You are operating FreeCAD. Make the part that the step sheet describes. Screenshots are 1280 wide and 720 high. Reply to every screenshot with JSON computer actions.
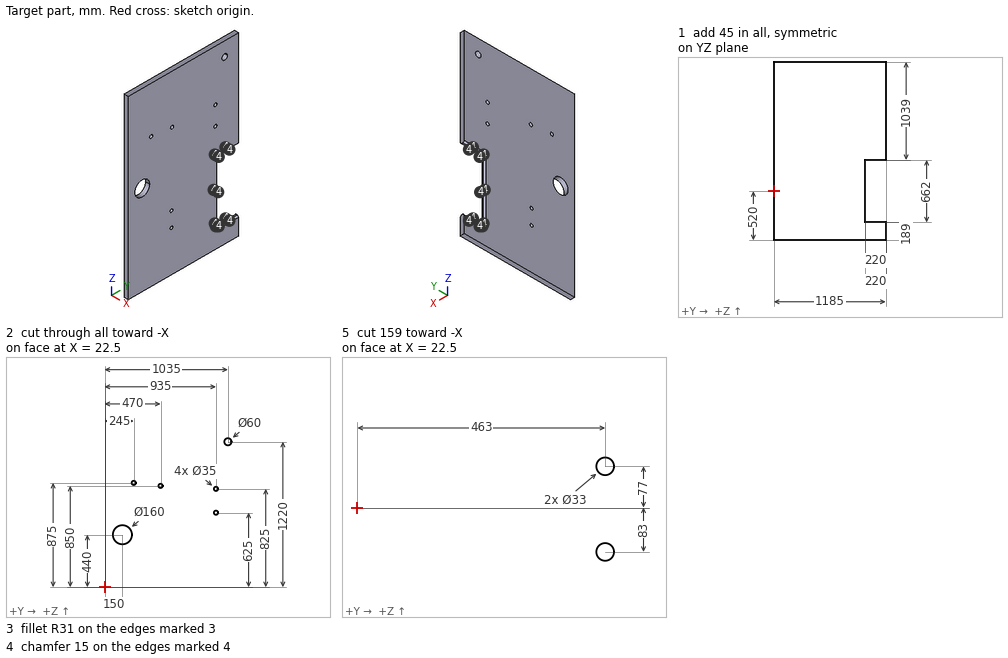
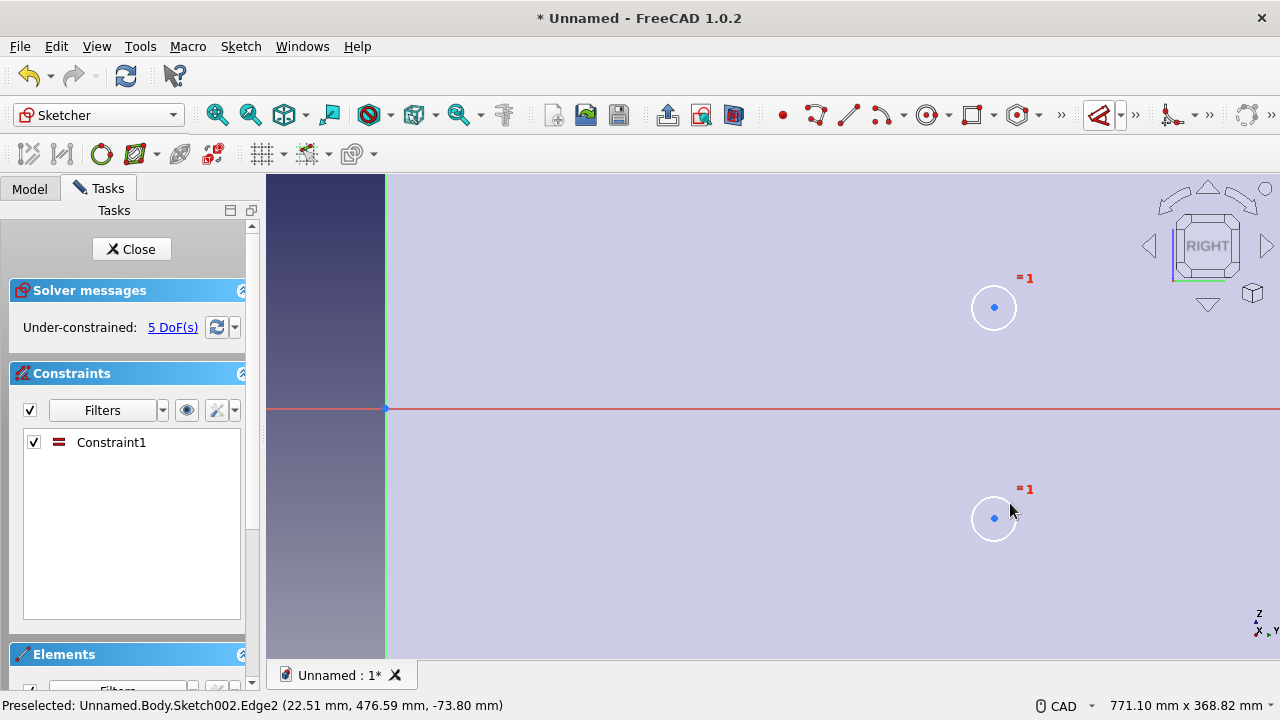
{"action": "left_click", "coordinate": [994, 308]}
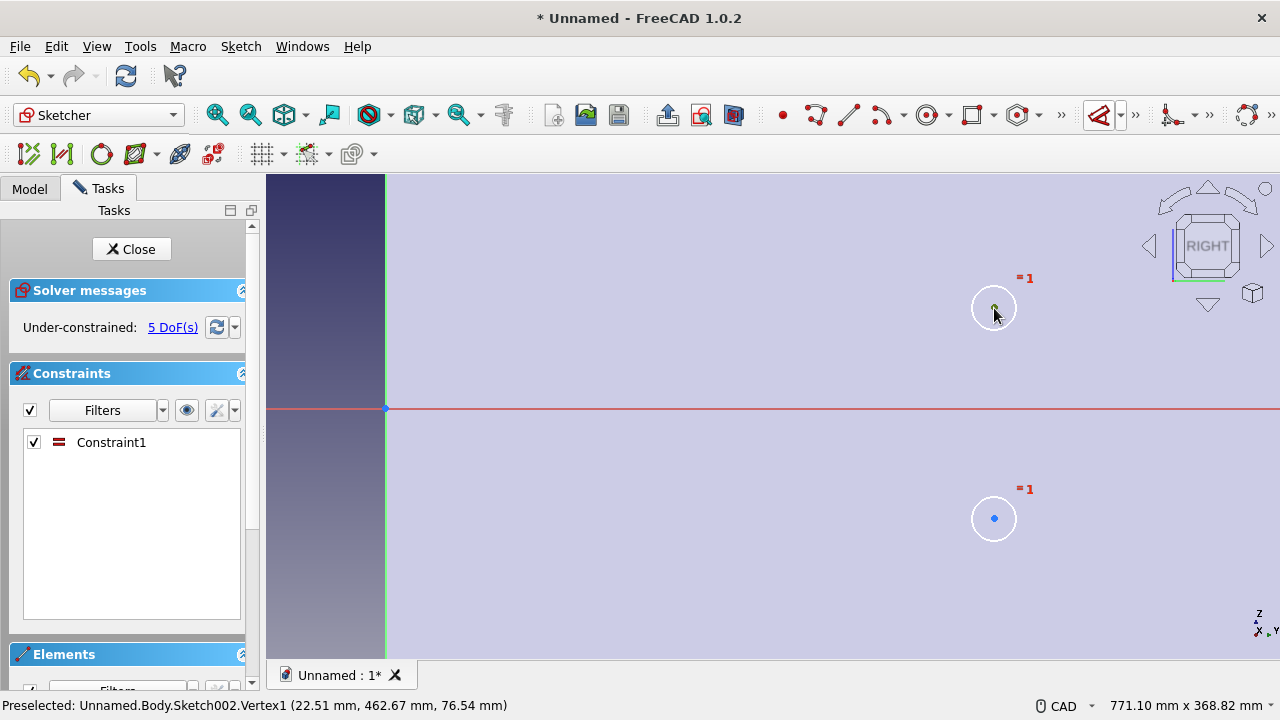
{"action": "left_click", "coordinate": [994, 519]}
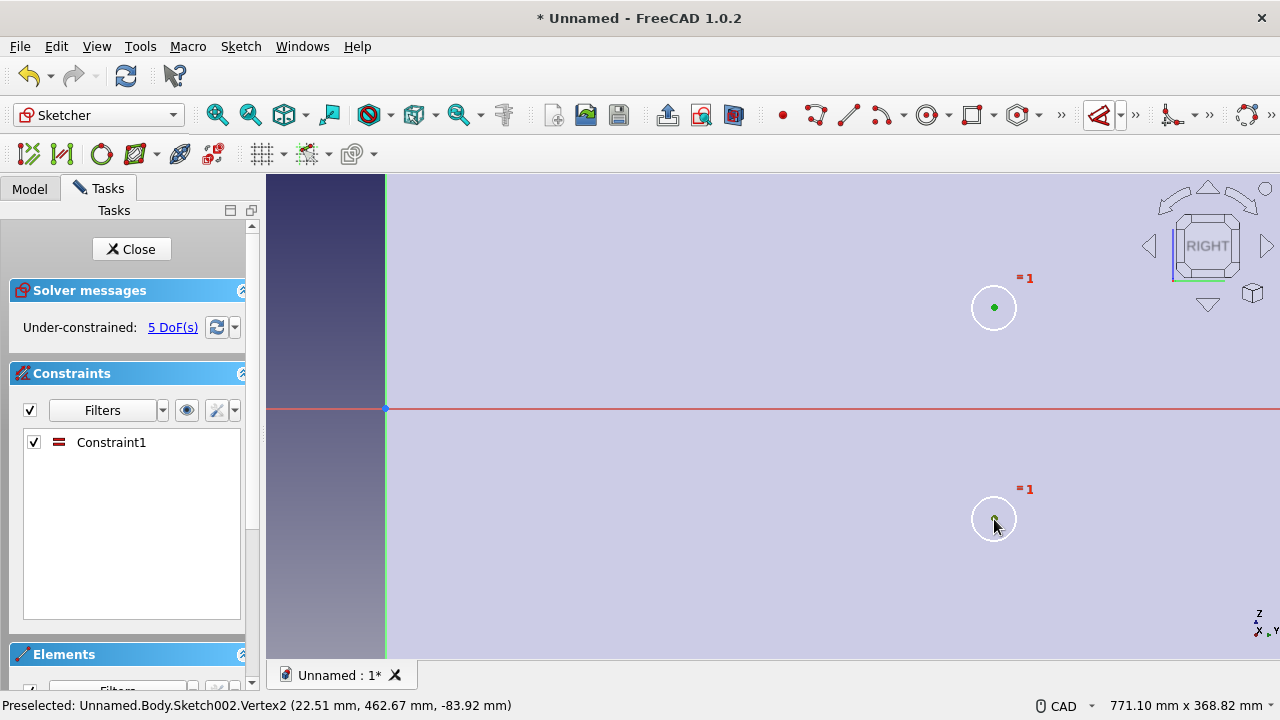
{"action": "key", "text": "v"}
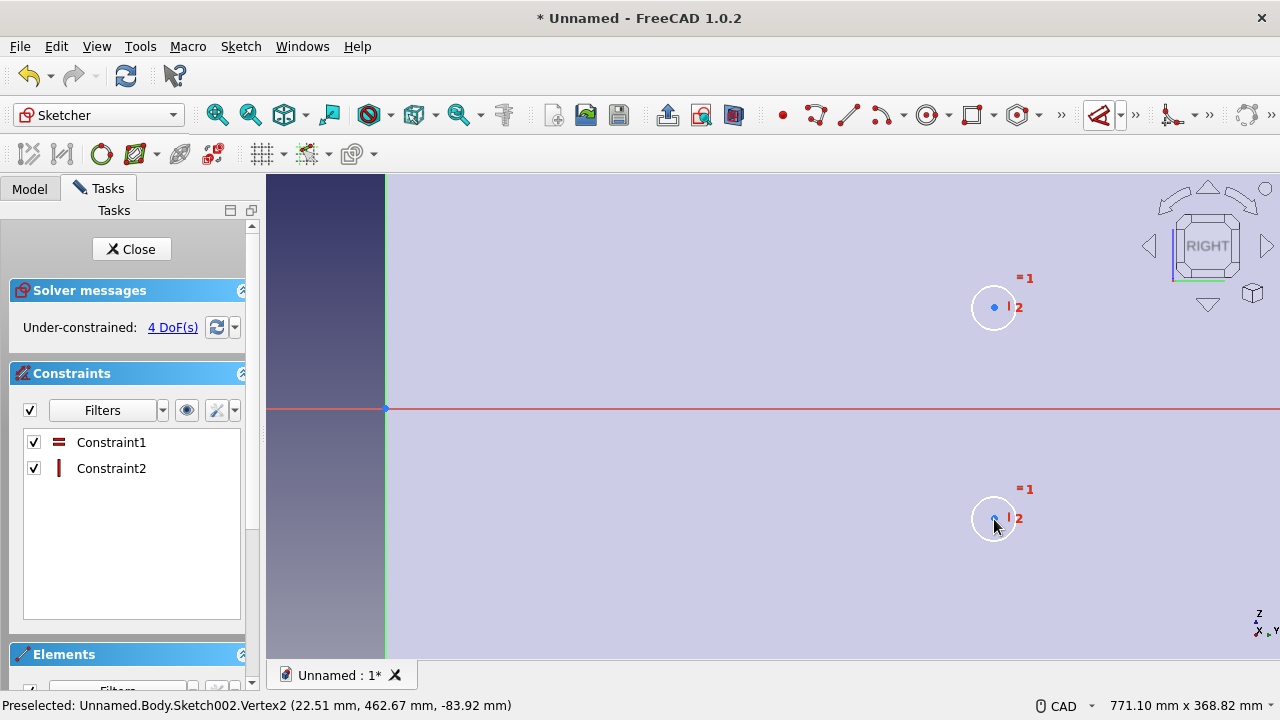
{"action": "left_click", "coordinate": [1009, 292]}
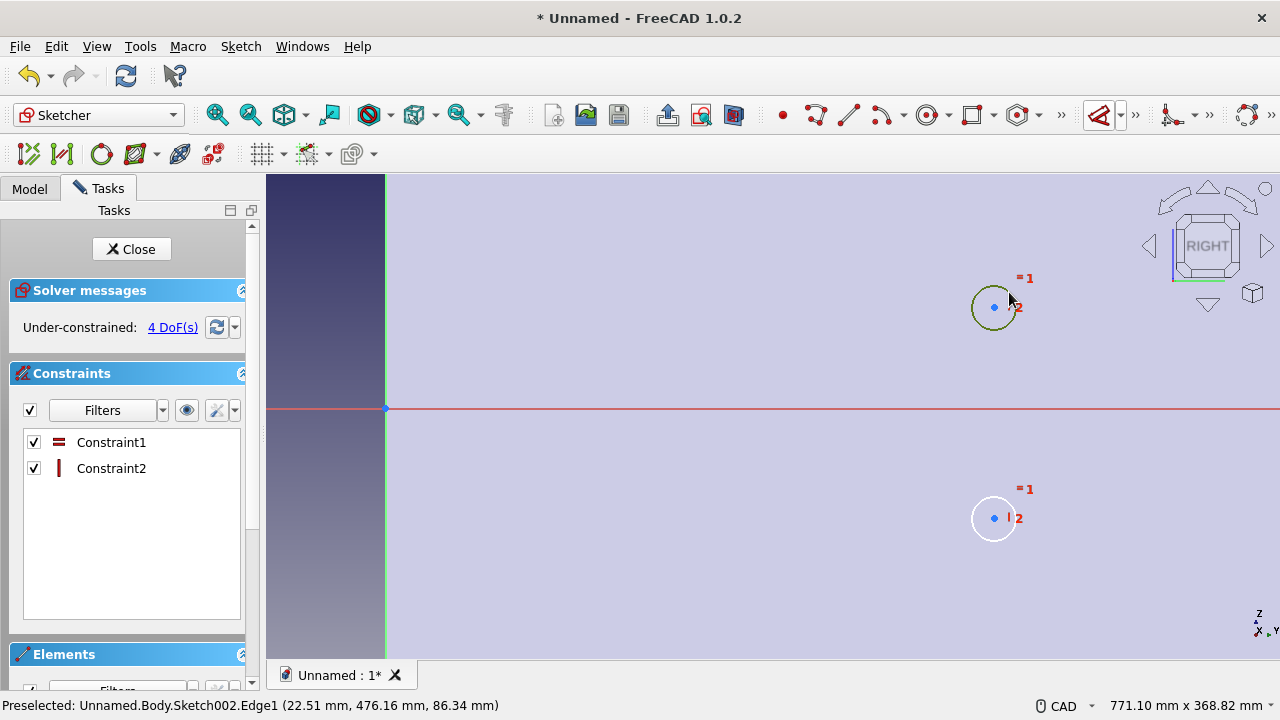
{"action": "key", "text": "k o"}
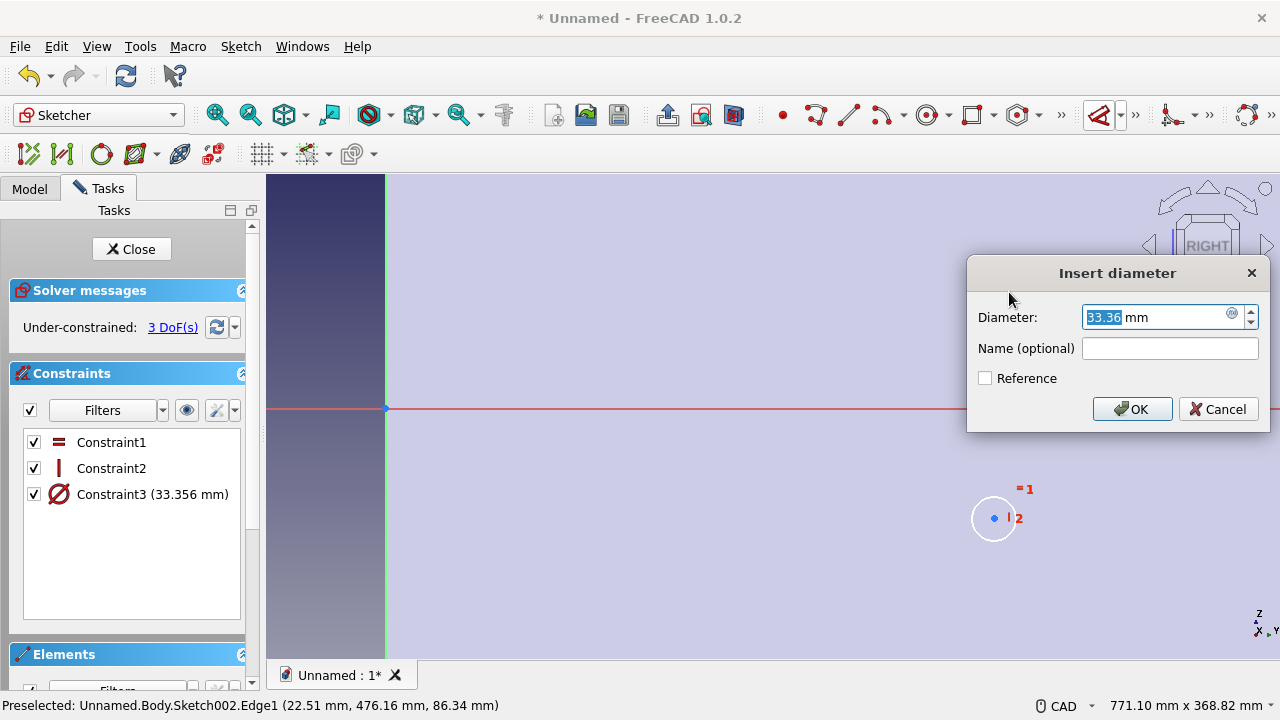
{"action": "type", "text": "33"}
{"action": "key", "text": "Return"}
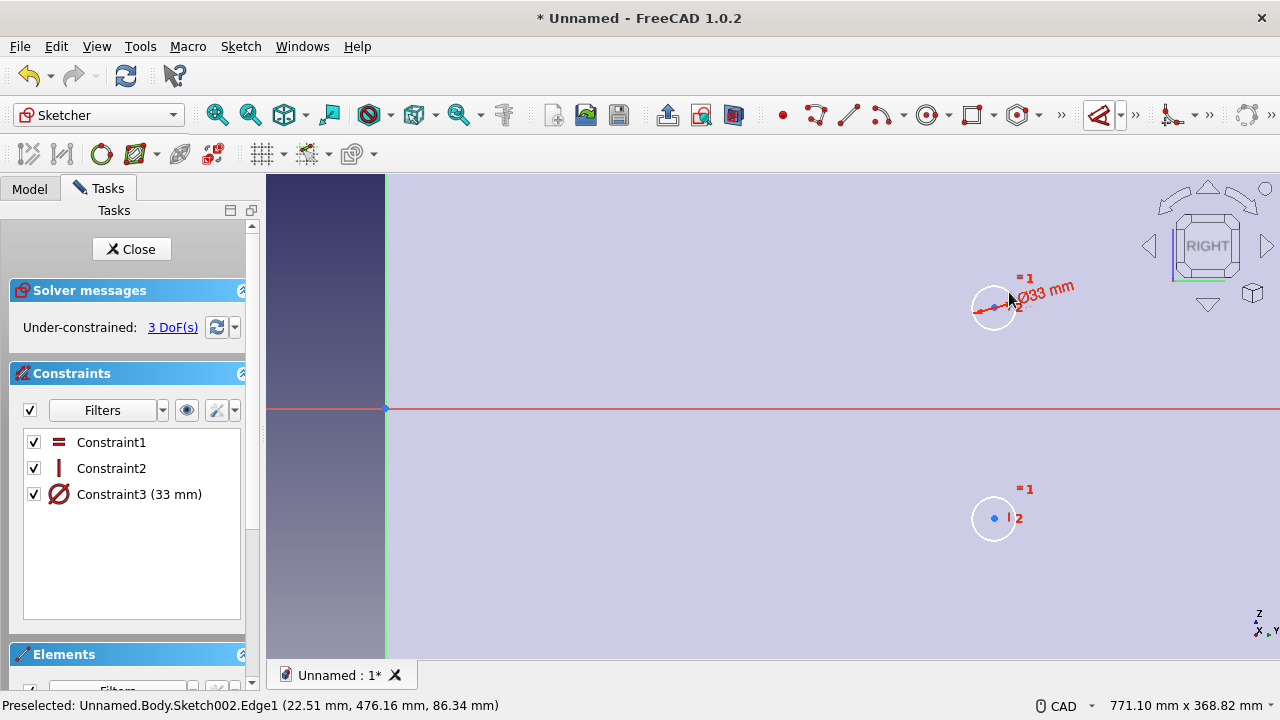
{"action": "left_click", "coordinate": [994, 308]}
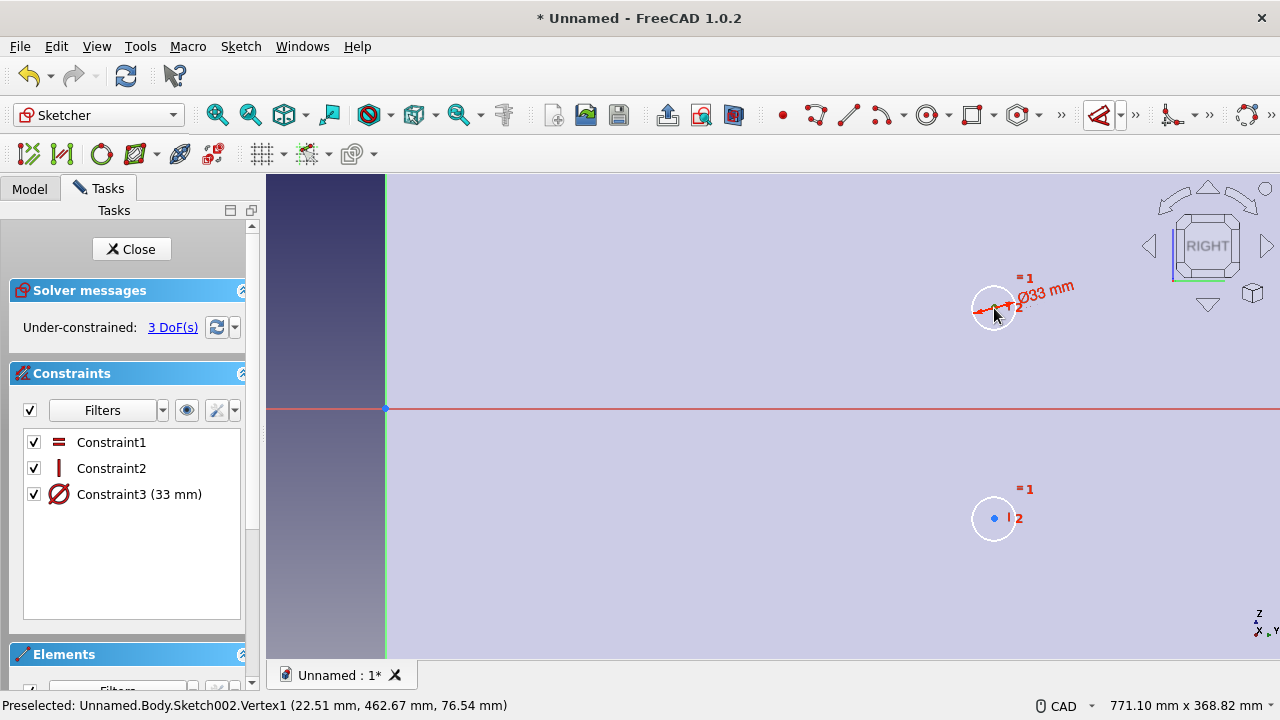
{"action": "key", "text": "i"}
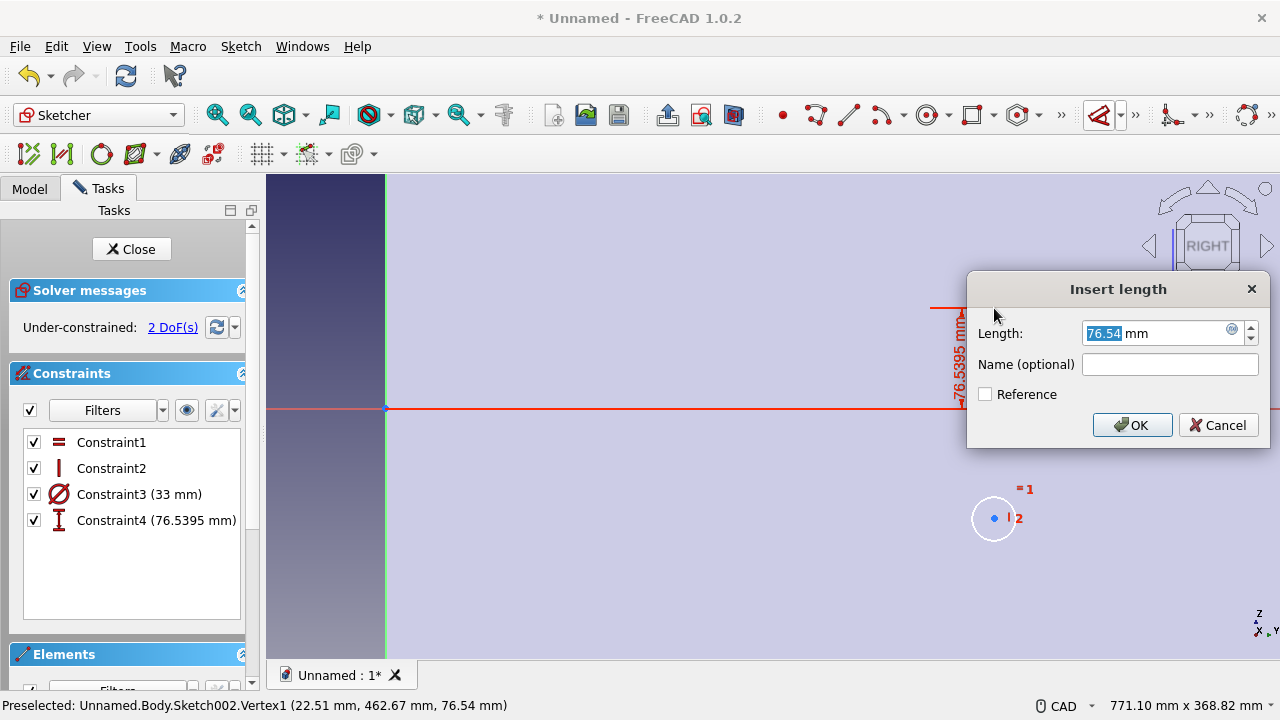
{"action": "type", "text": "77"}
{"action": "key", "text": "Return"}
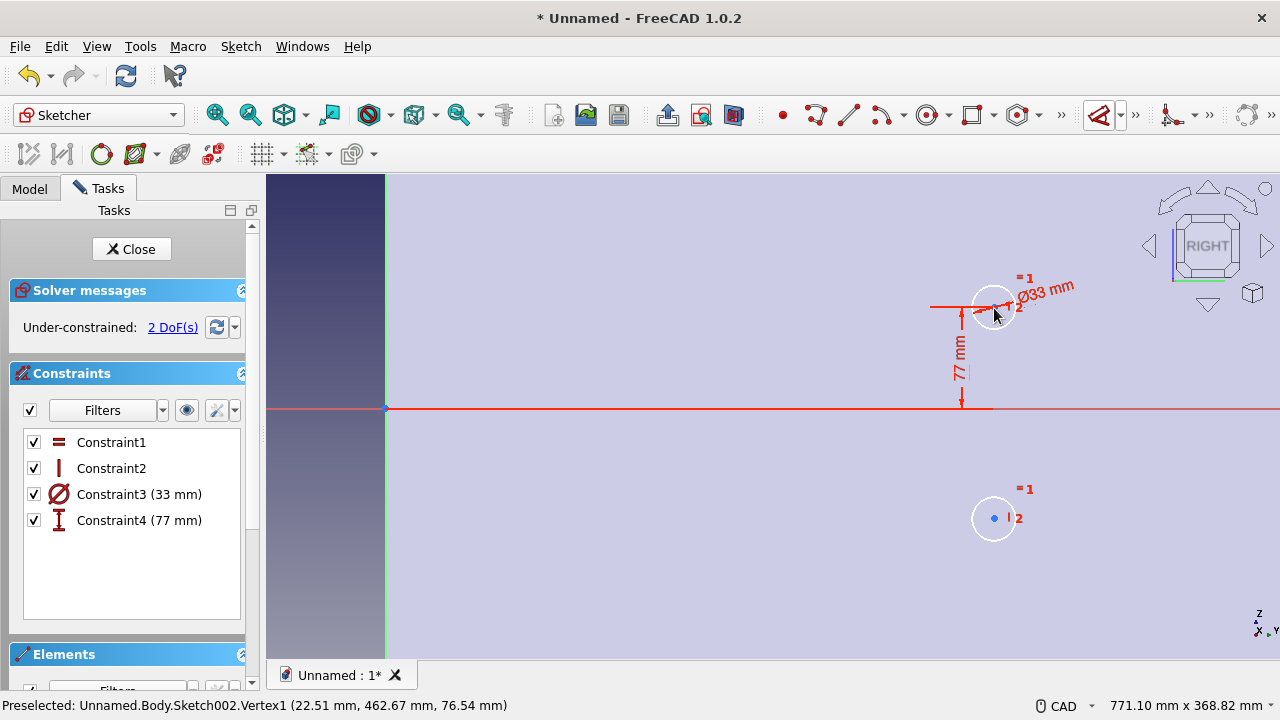
{"action": "left_click", "coordinate": [994, 519]}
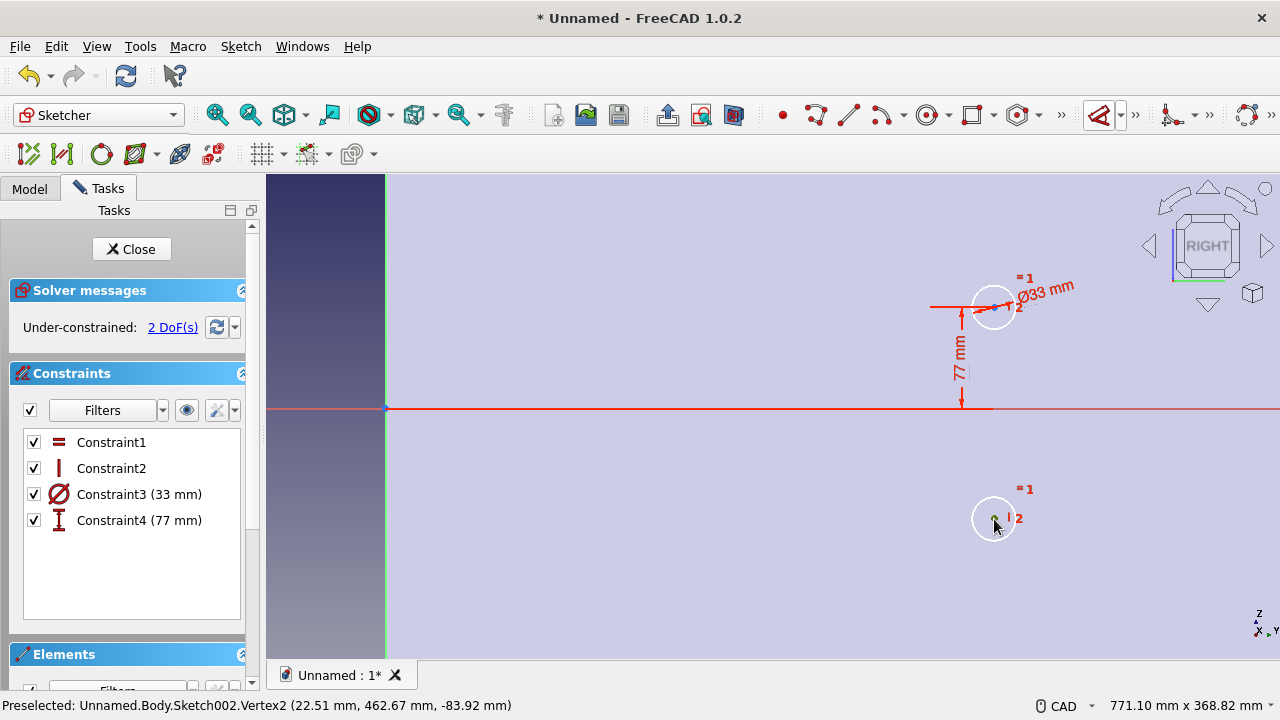
{"action": "key", "text": "i"}